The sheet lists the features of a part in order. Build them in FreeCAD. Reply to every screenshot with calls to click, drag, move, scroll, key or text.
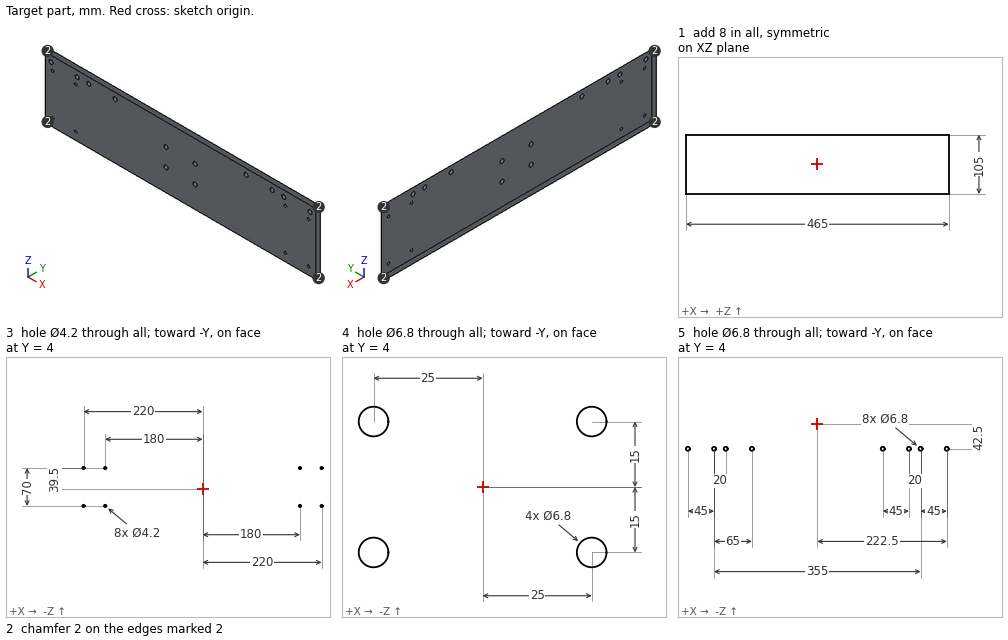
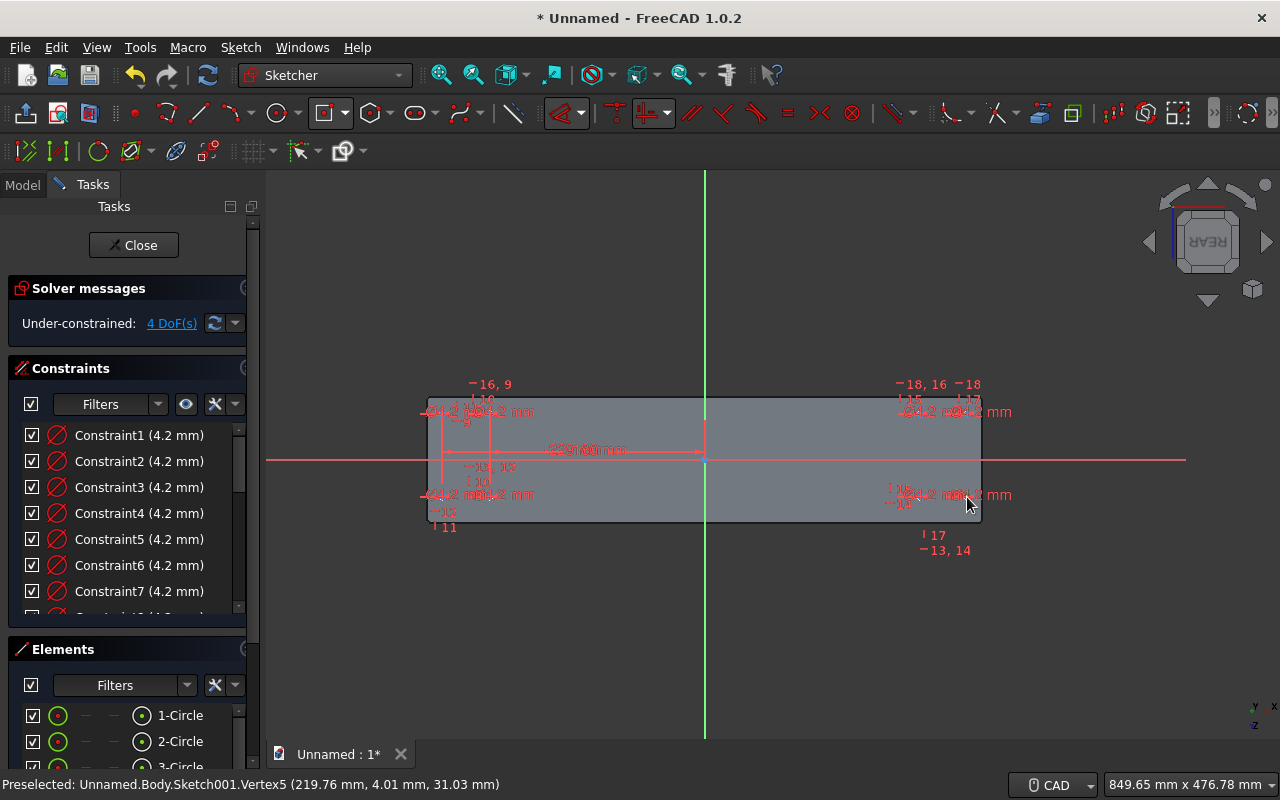
key(l)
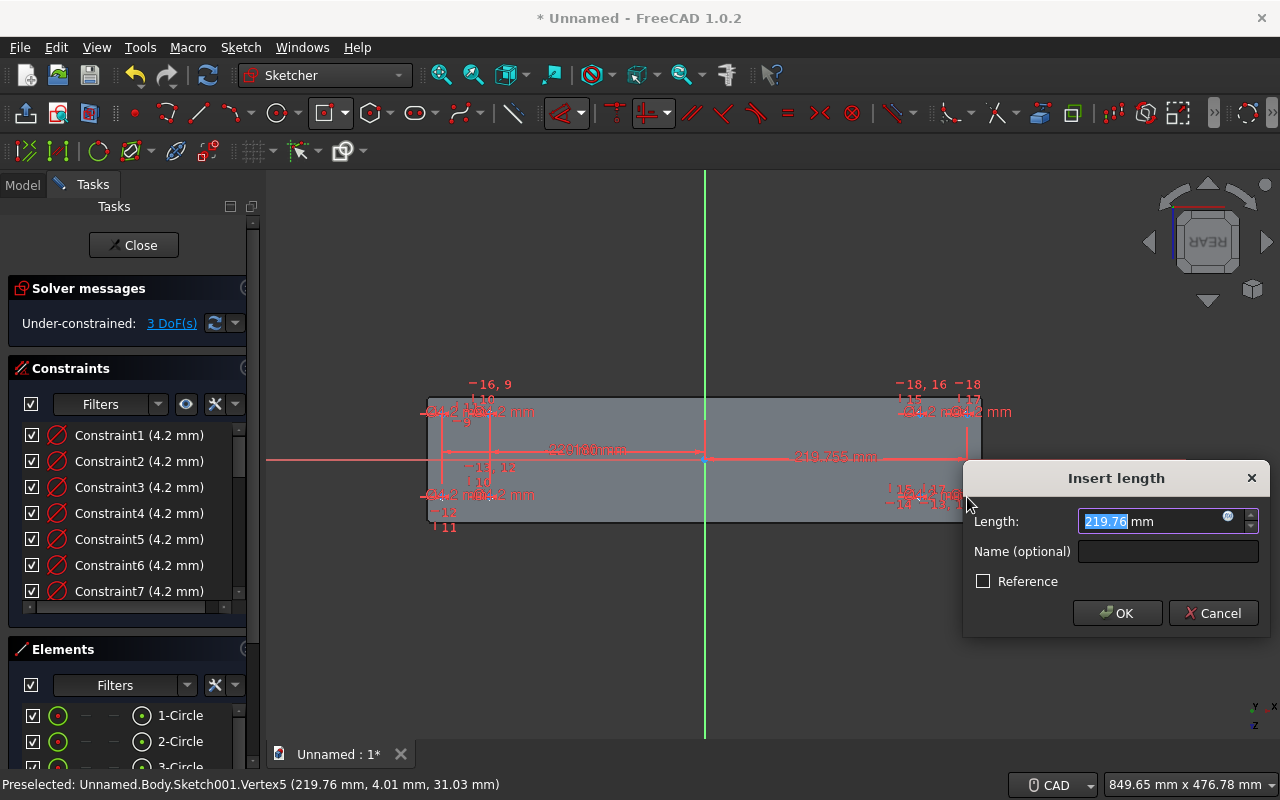
text(220)
key(Return)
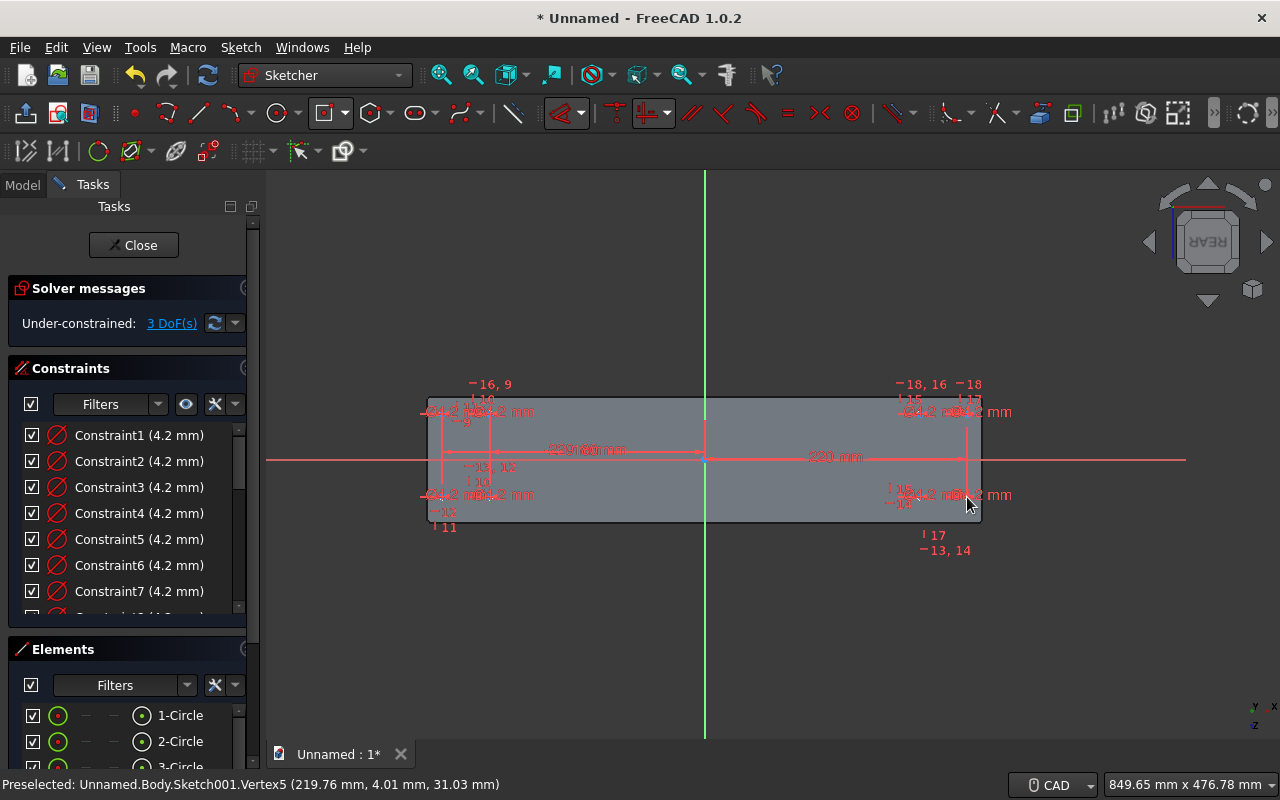
click(920, 497)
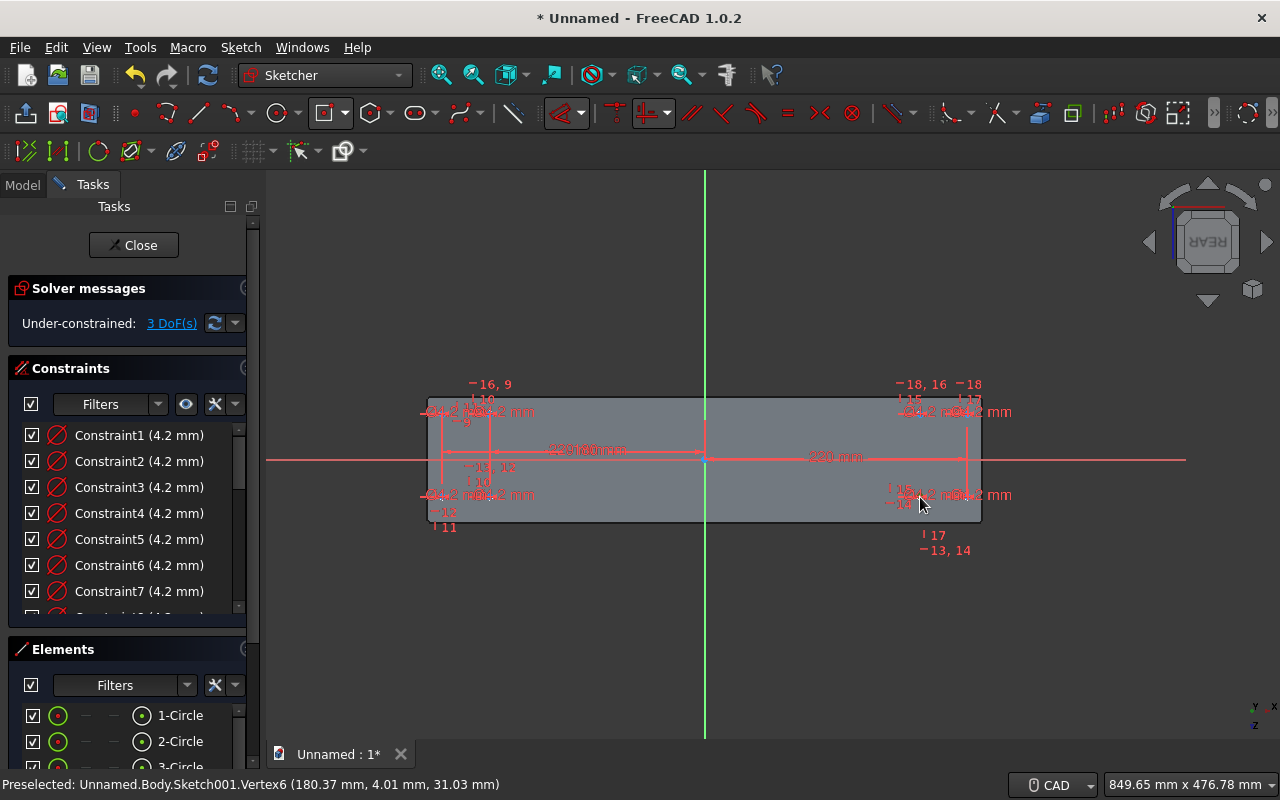
key(l)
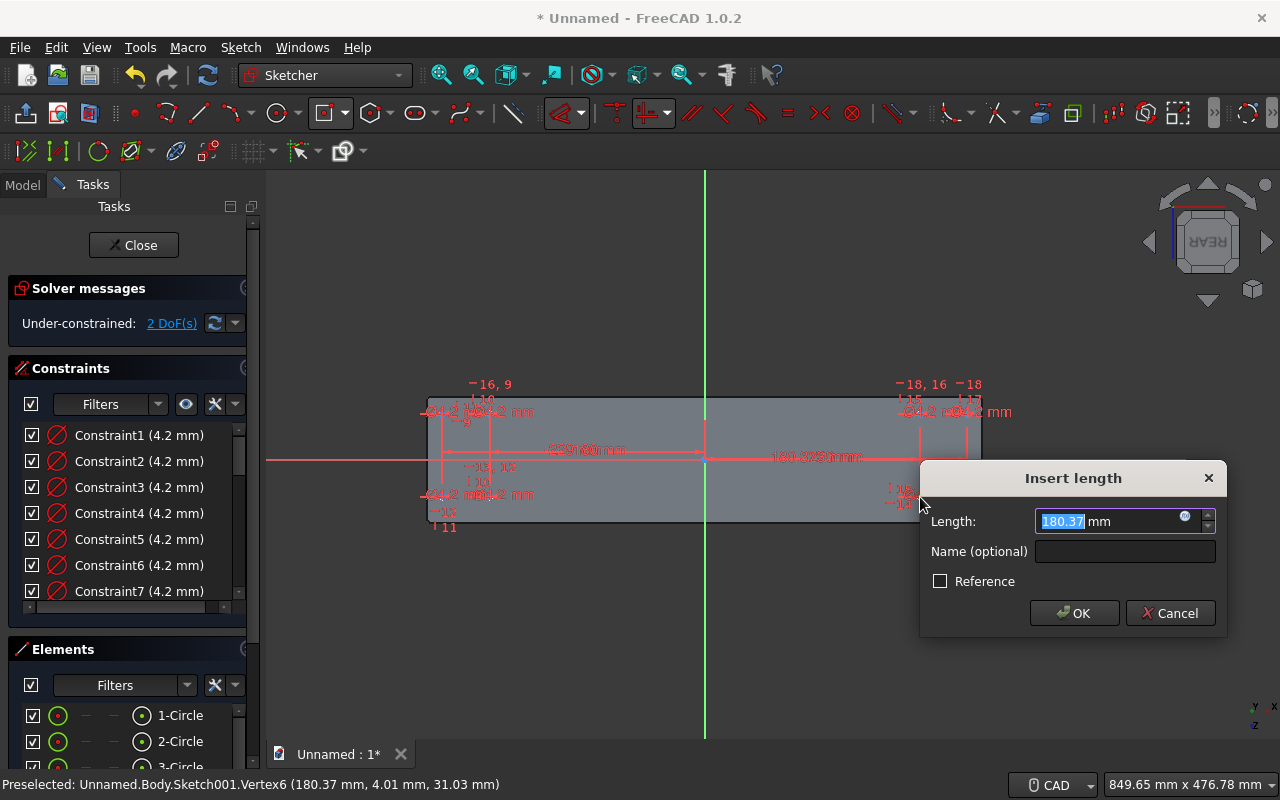
text(180)
key(Return)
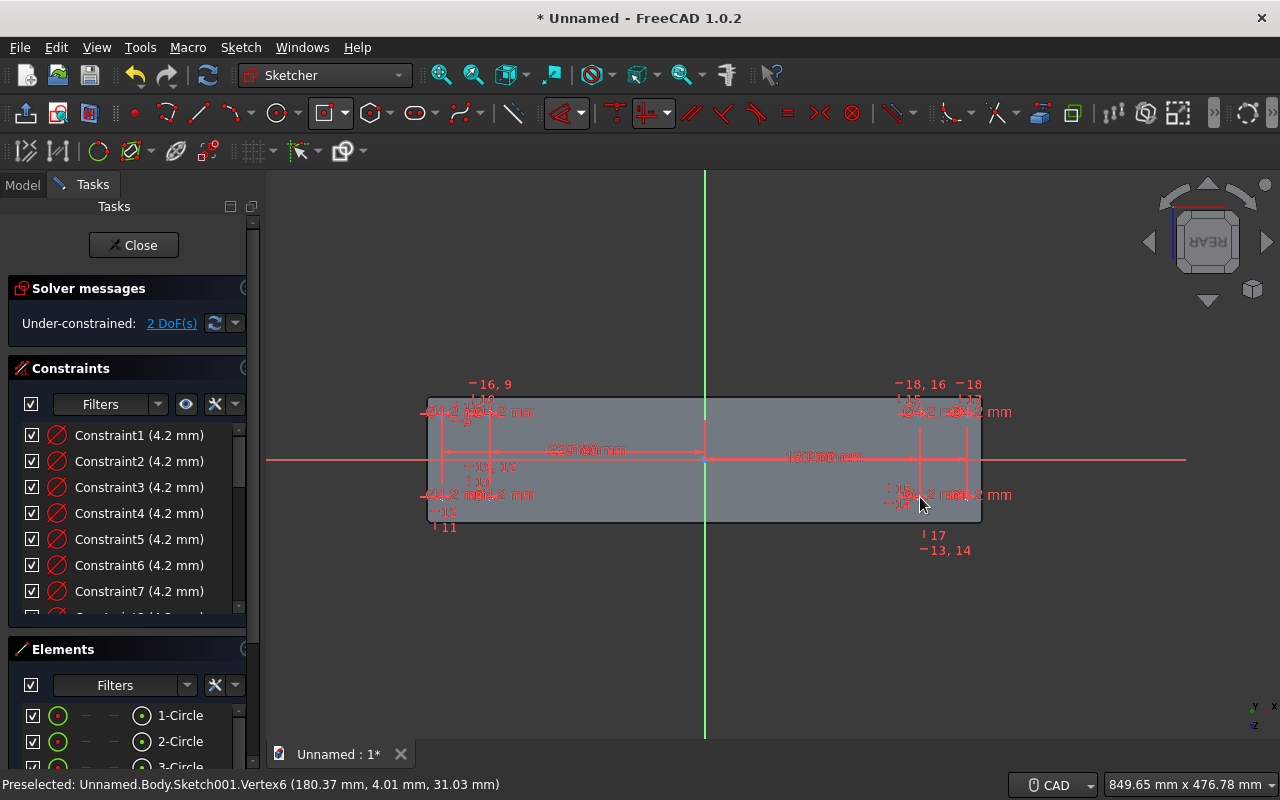
click(490, 414)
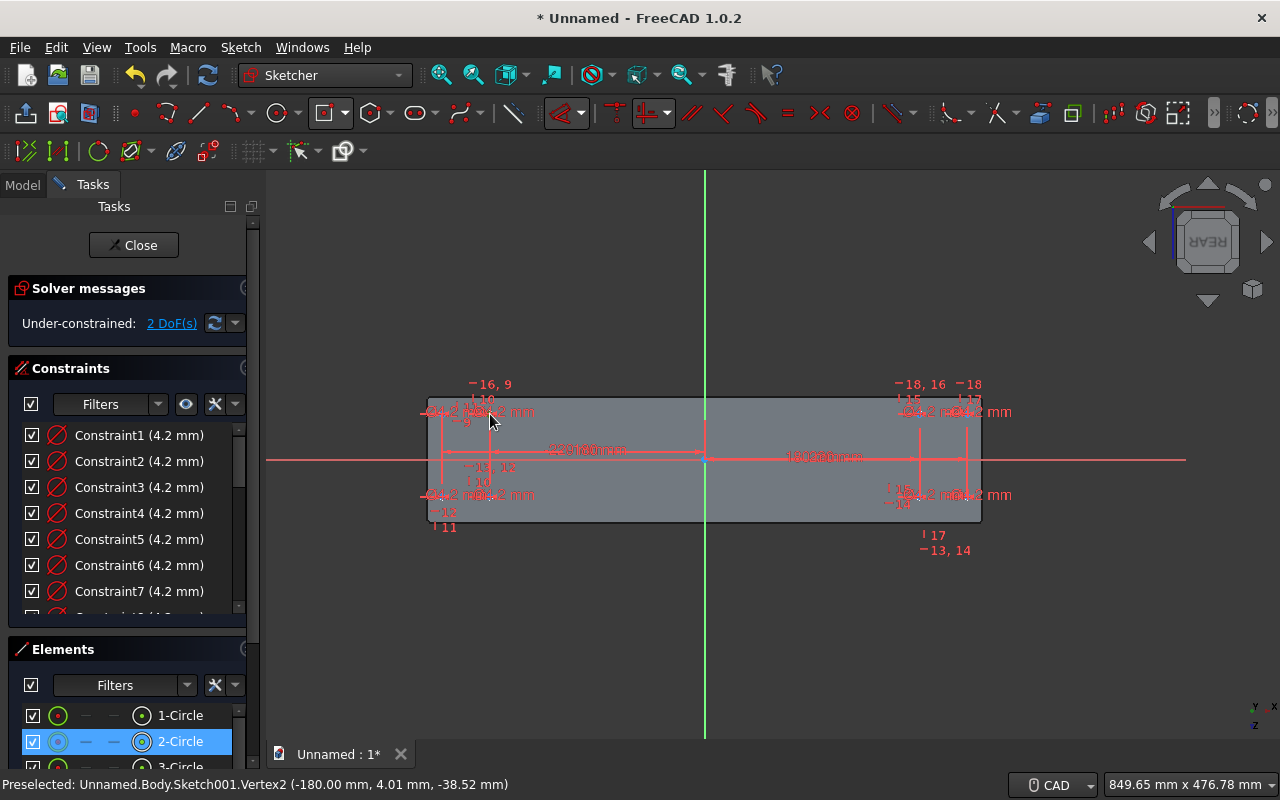
click(490, 497)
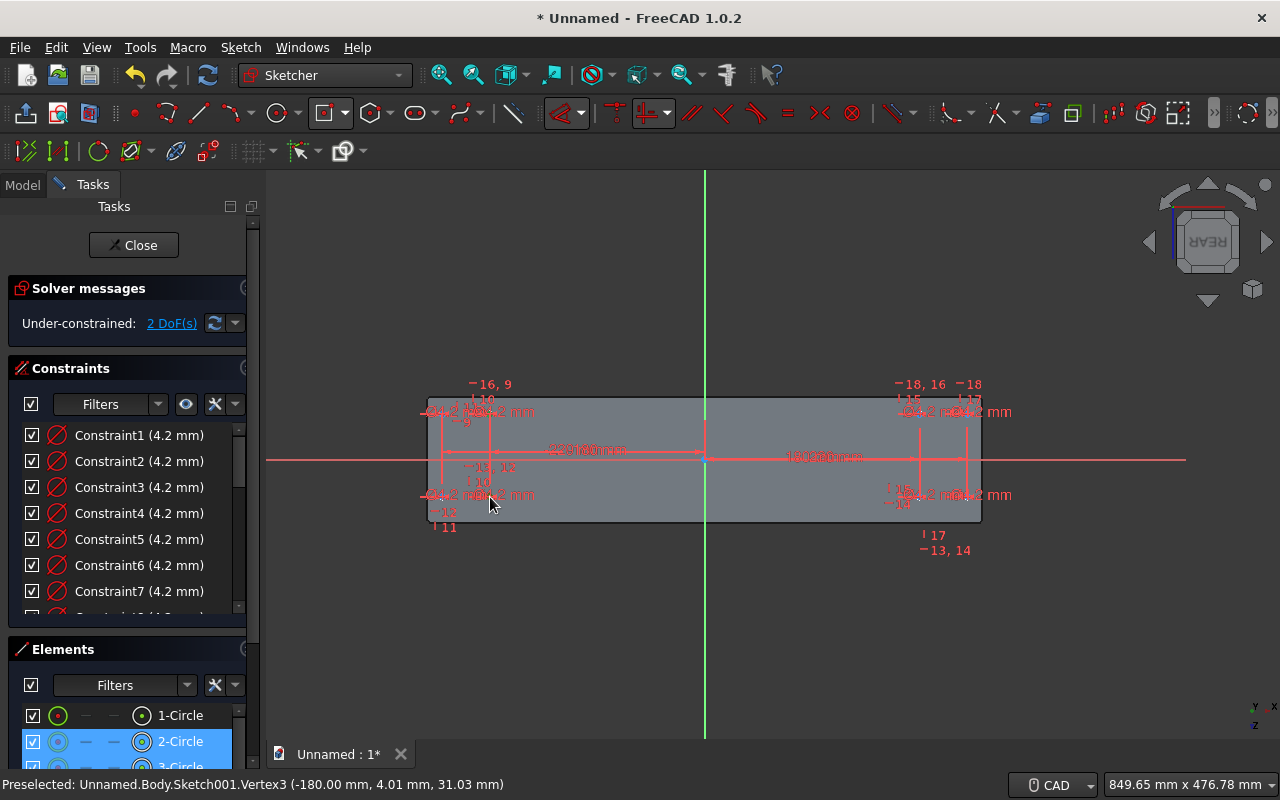
click(584, 114)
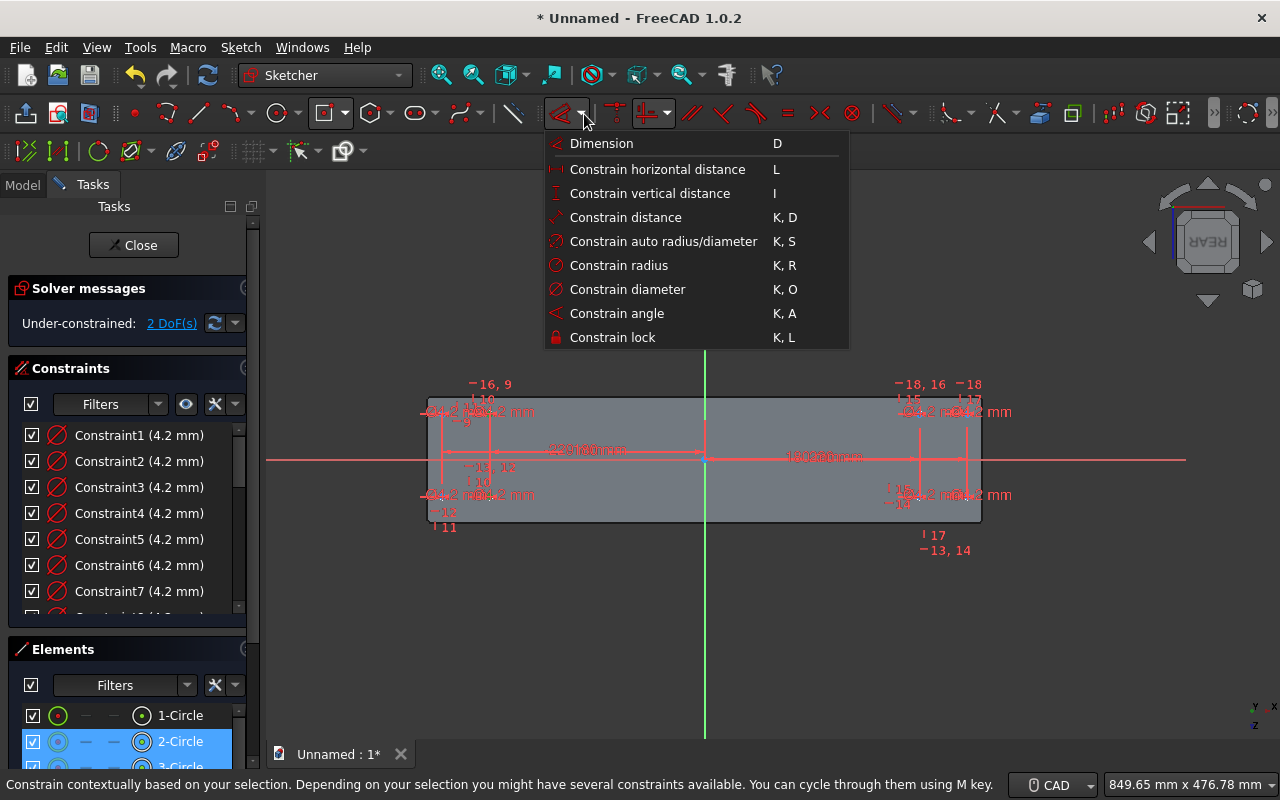
click(697, 193)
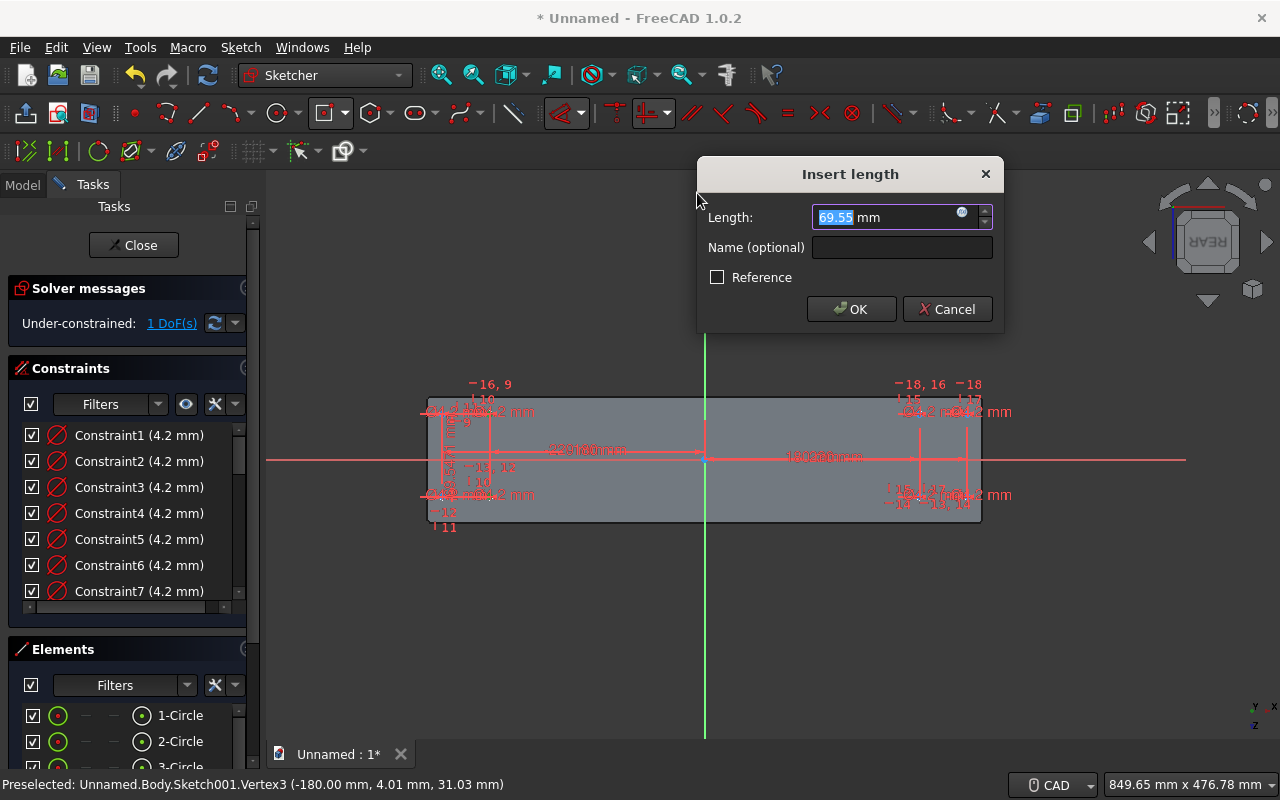
text(70)
key(Return)